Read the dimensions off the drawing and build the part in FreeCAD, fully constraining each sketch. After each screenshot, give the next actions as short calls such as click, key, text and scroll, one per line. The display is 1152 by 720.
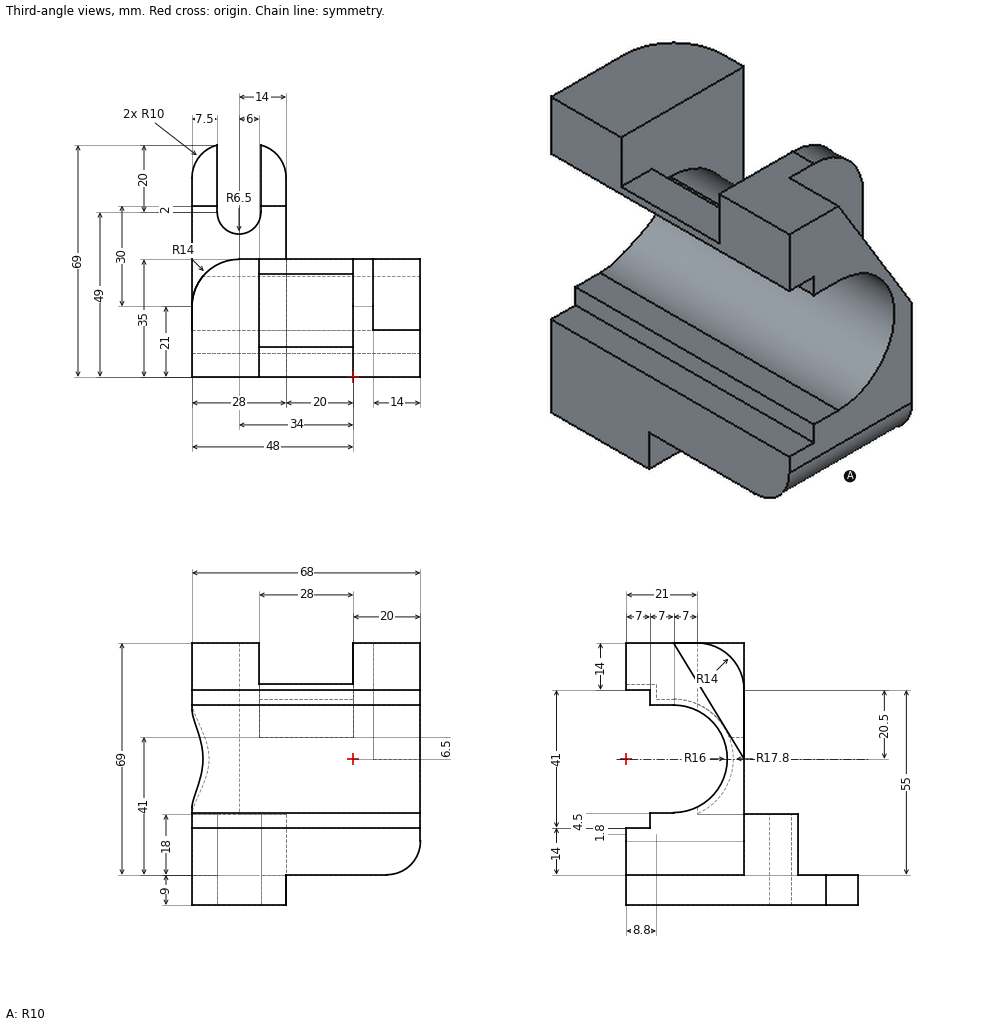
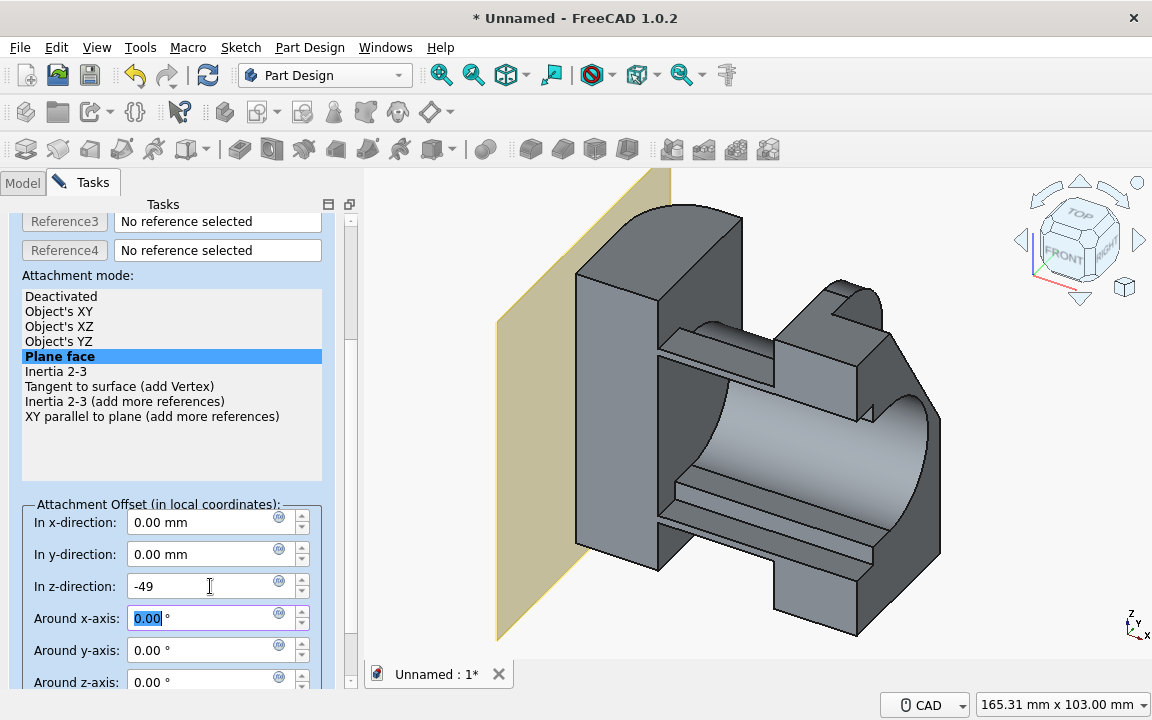
scroll(351, 451, up, 4)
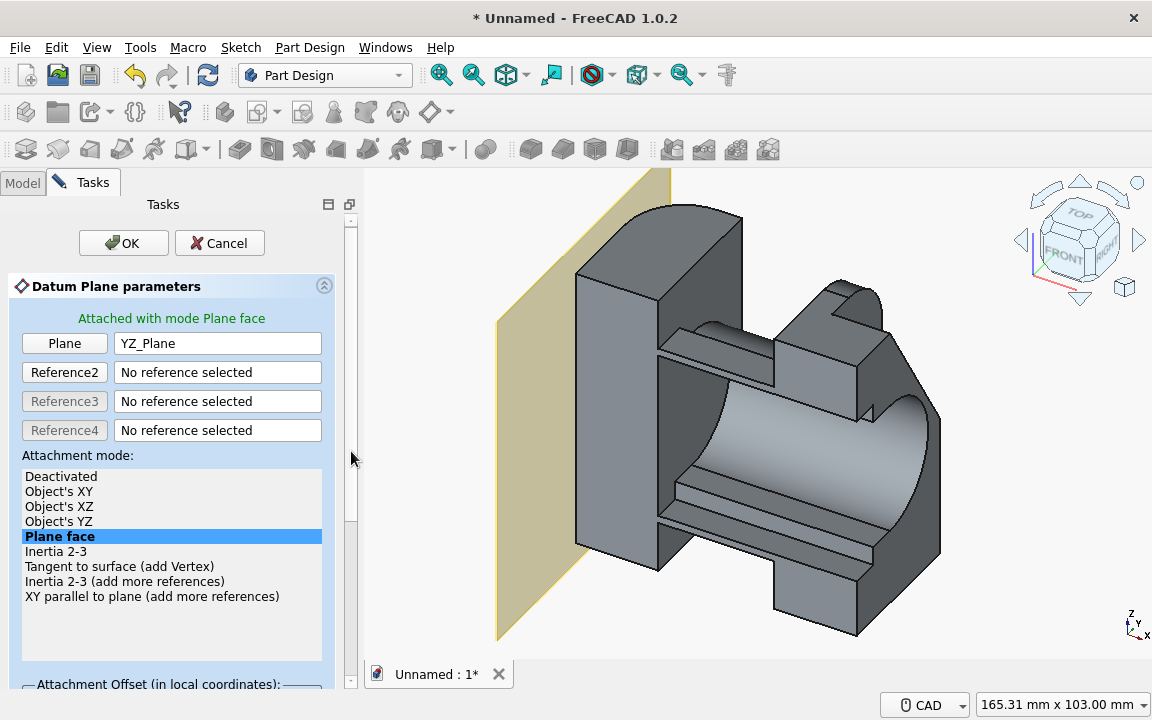
click(124, 243)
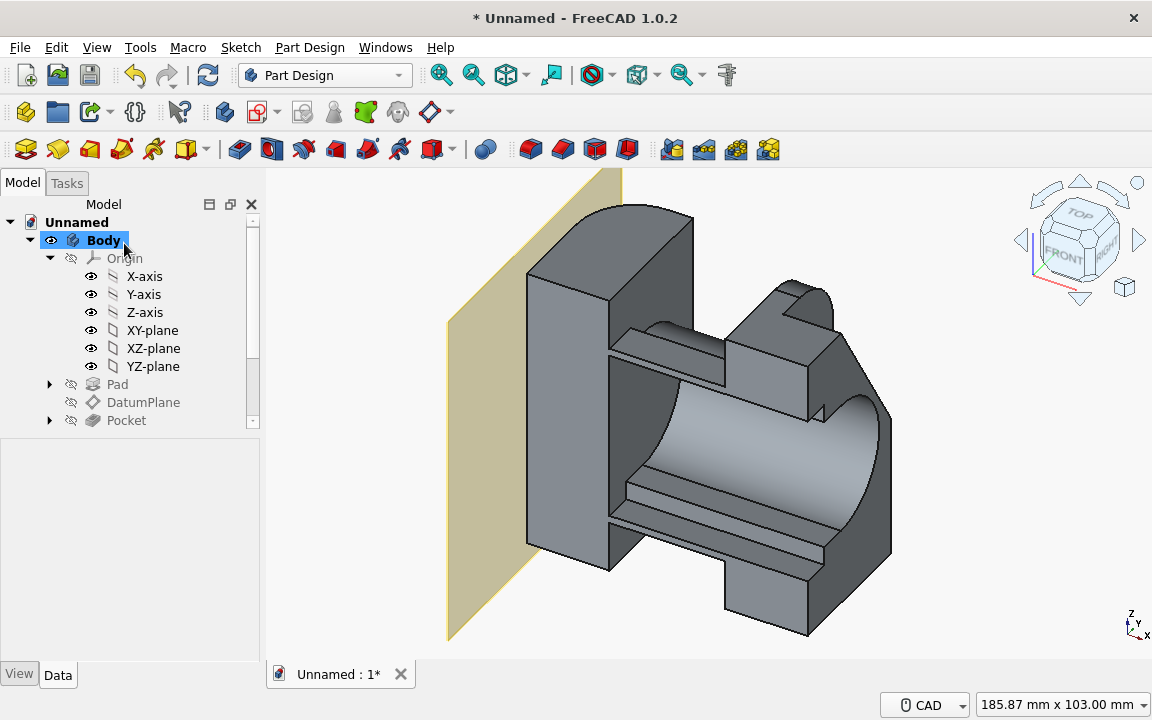
scroll(100, 326, down, 3)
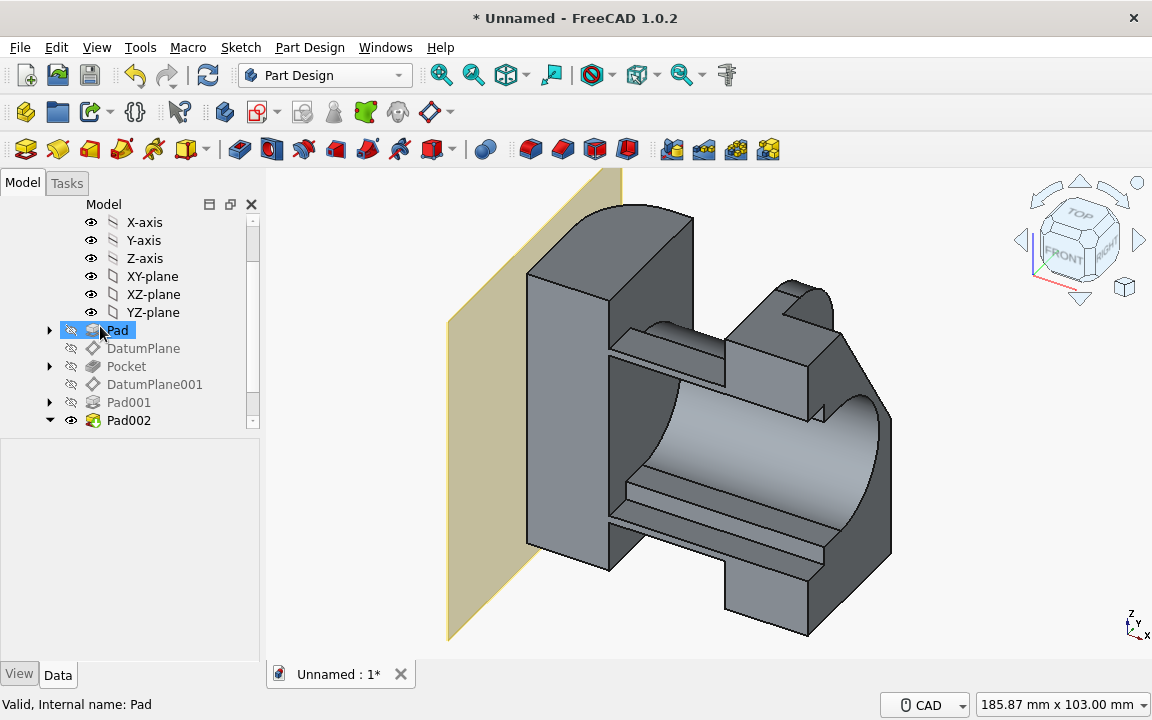
click(116, 420)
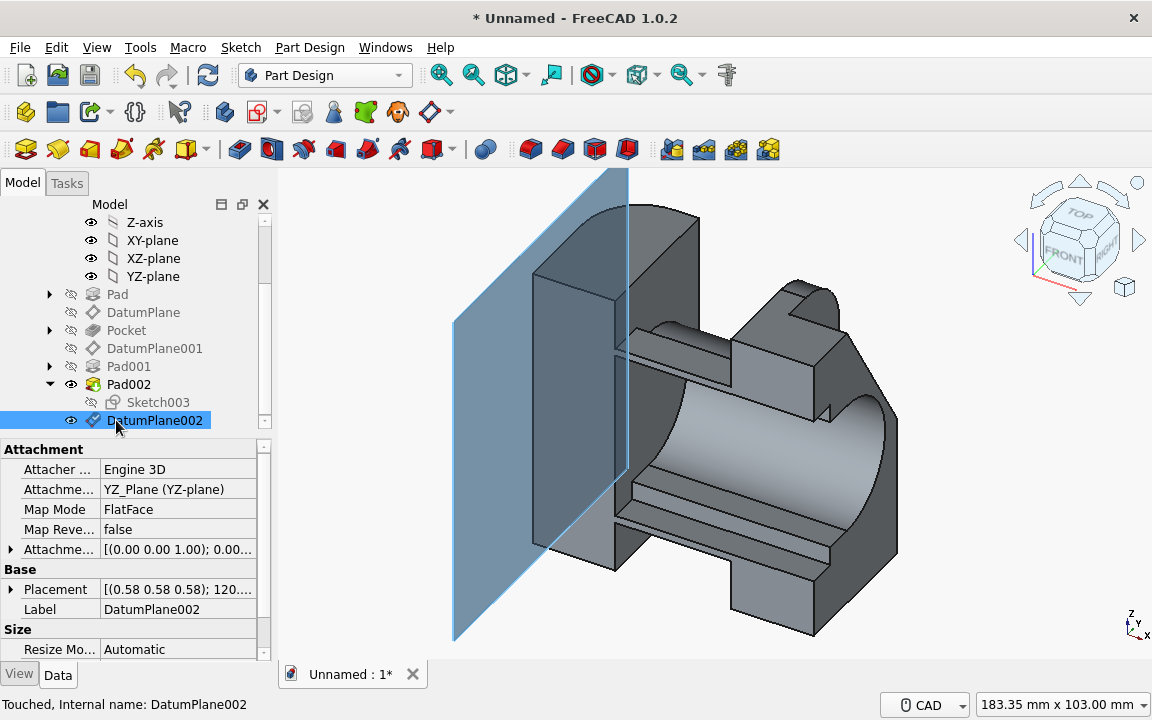
click(258, 112)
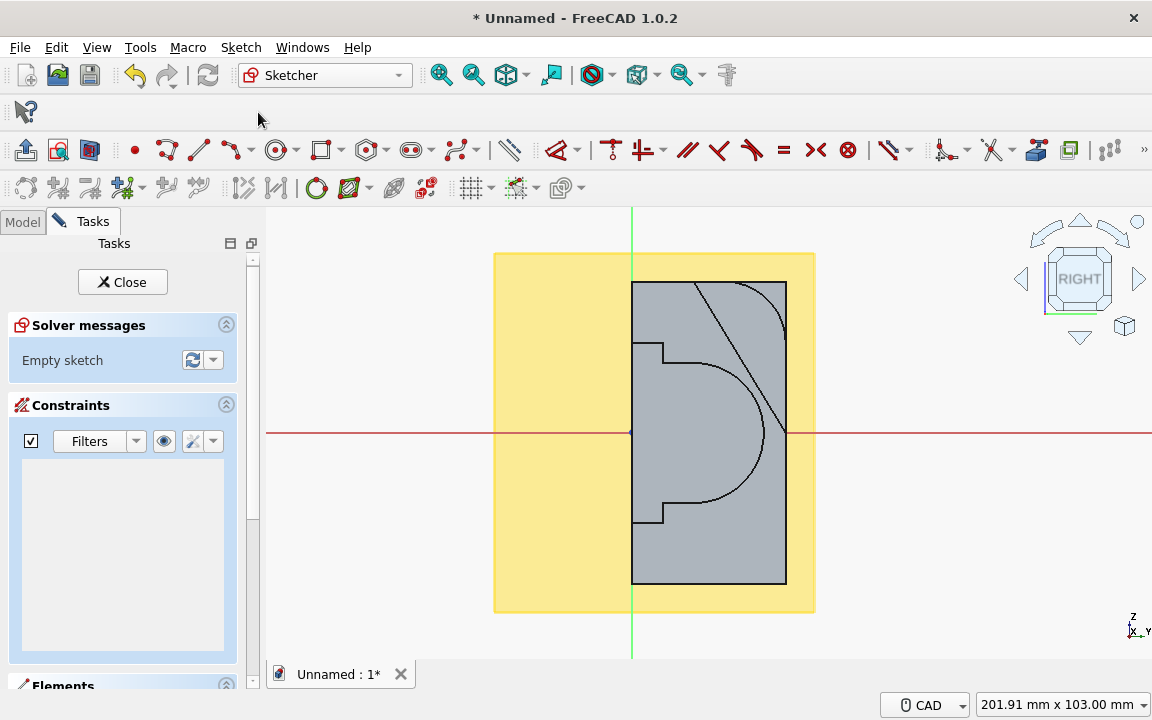
click(90, 150)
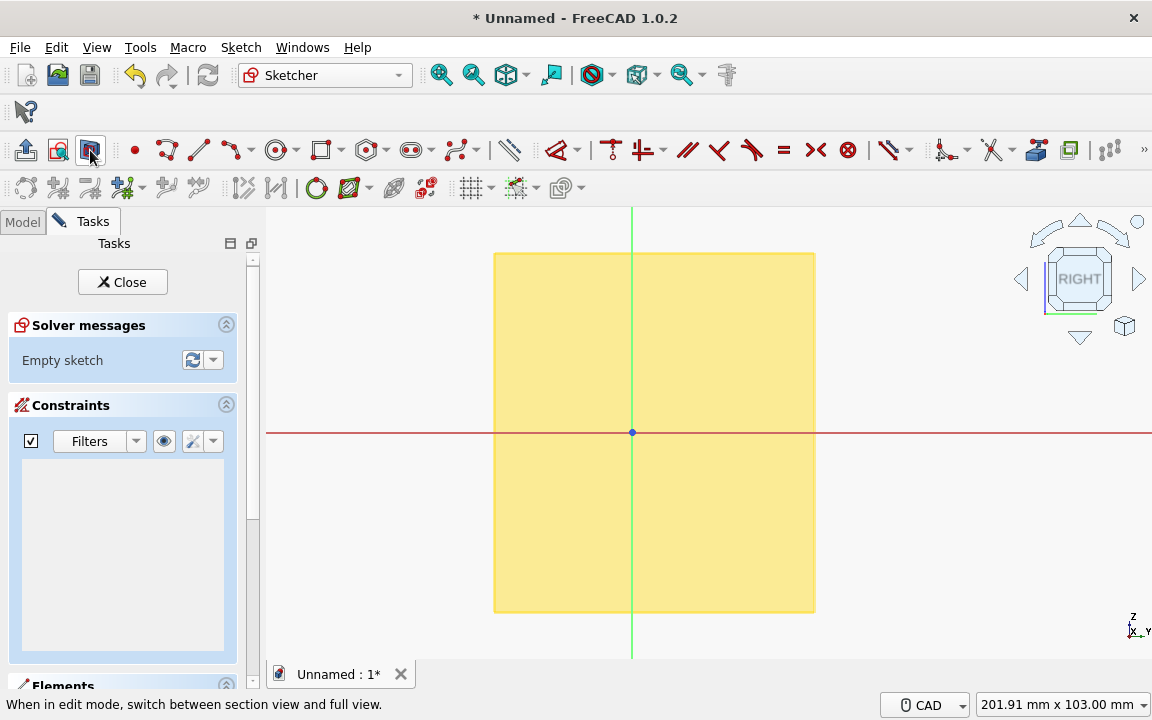
scroll(815, 433, up, 2)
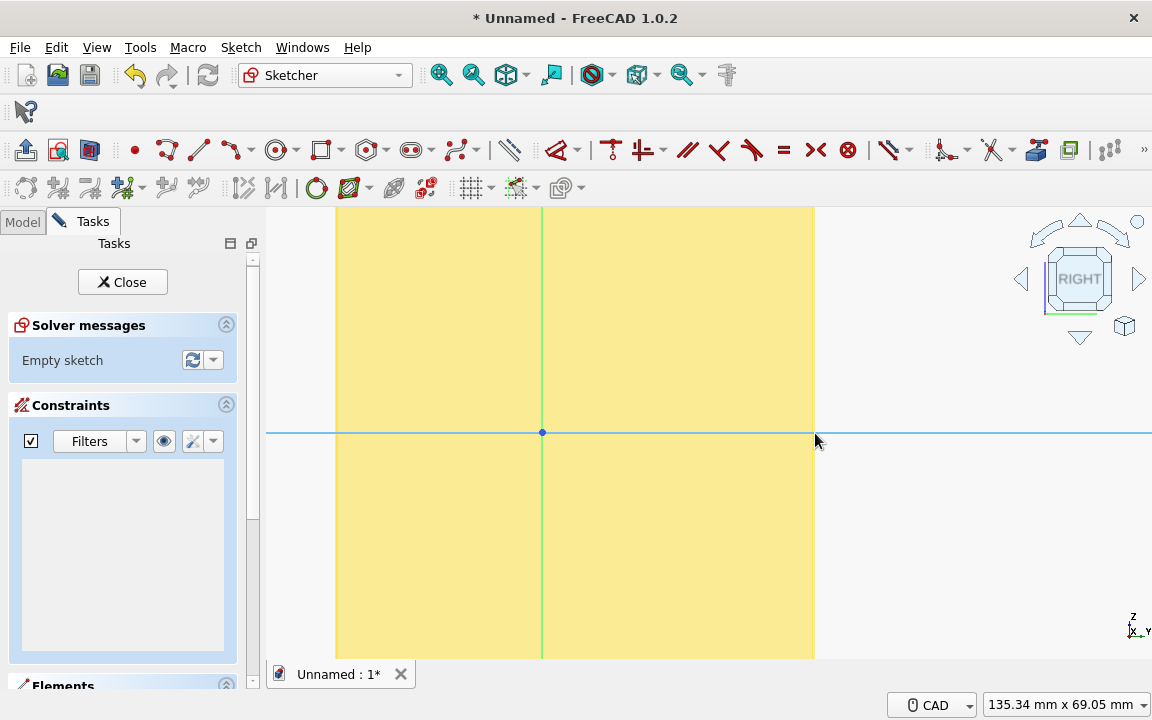
click(168, 150)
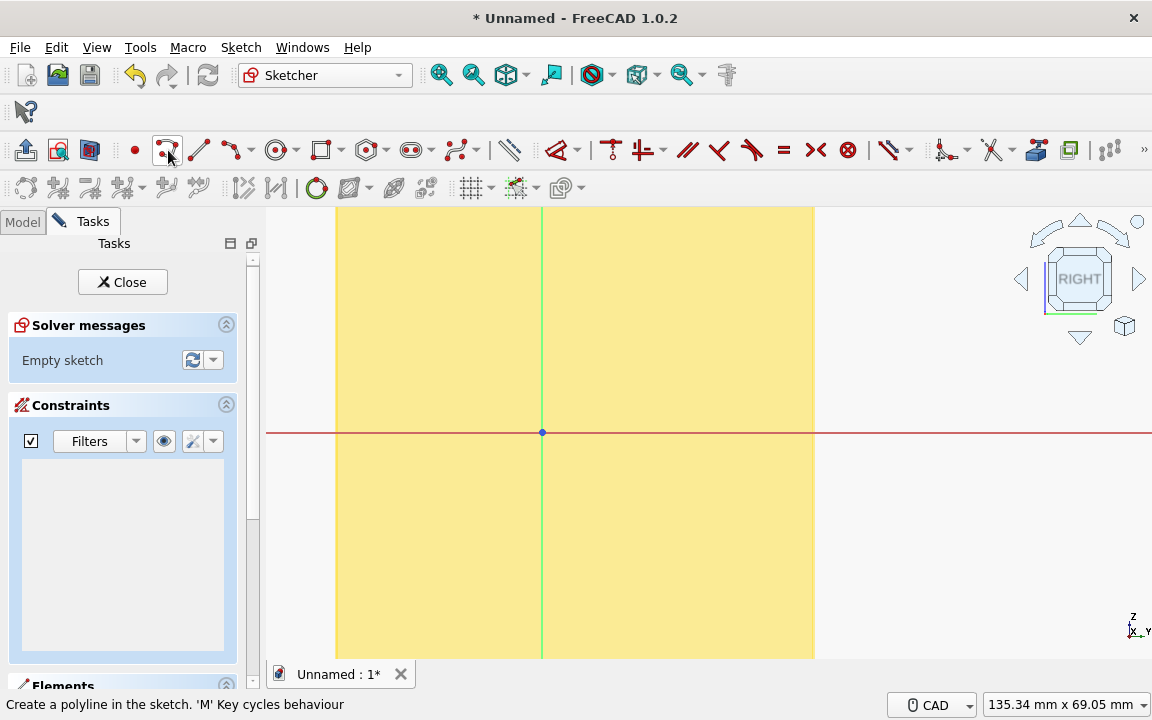
click(634, 328)
click(588, 328)
click(588, 299)
click(542, 299)
click(551, 567)
click(588, 567)
click(588, 537)
click(634, 537)
right_click(634, 537)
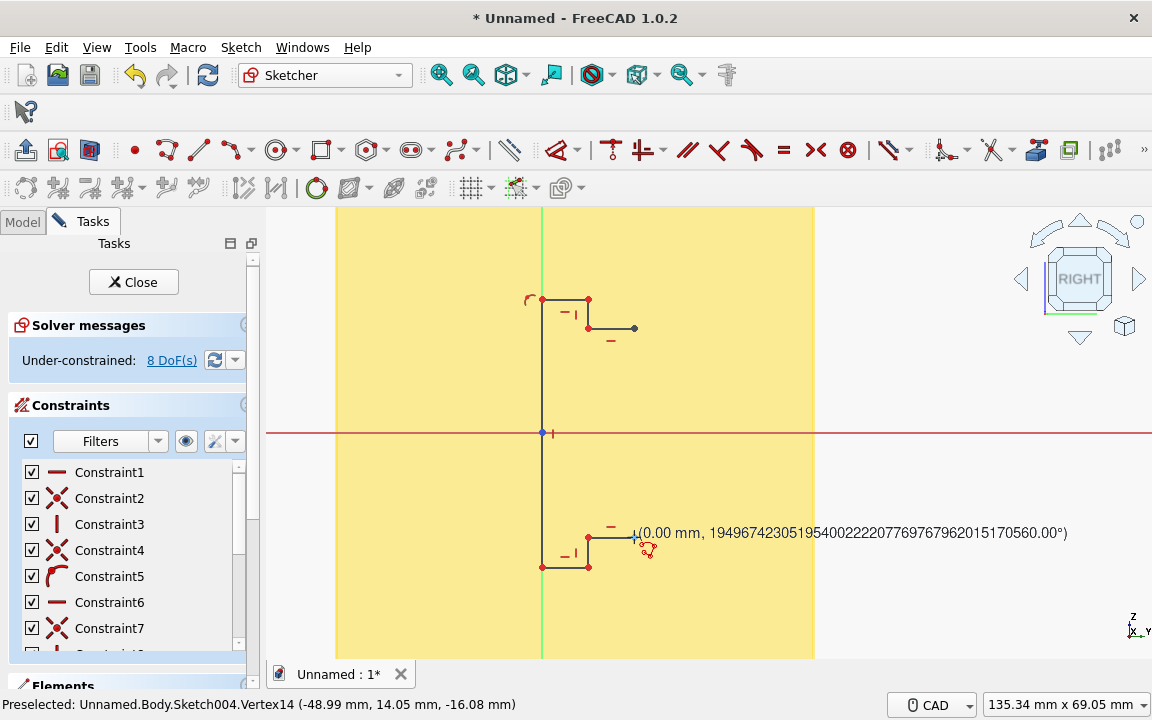
key(g)
key(3)
key(a)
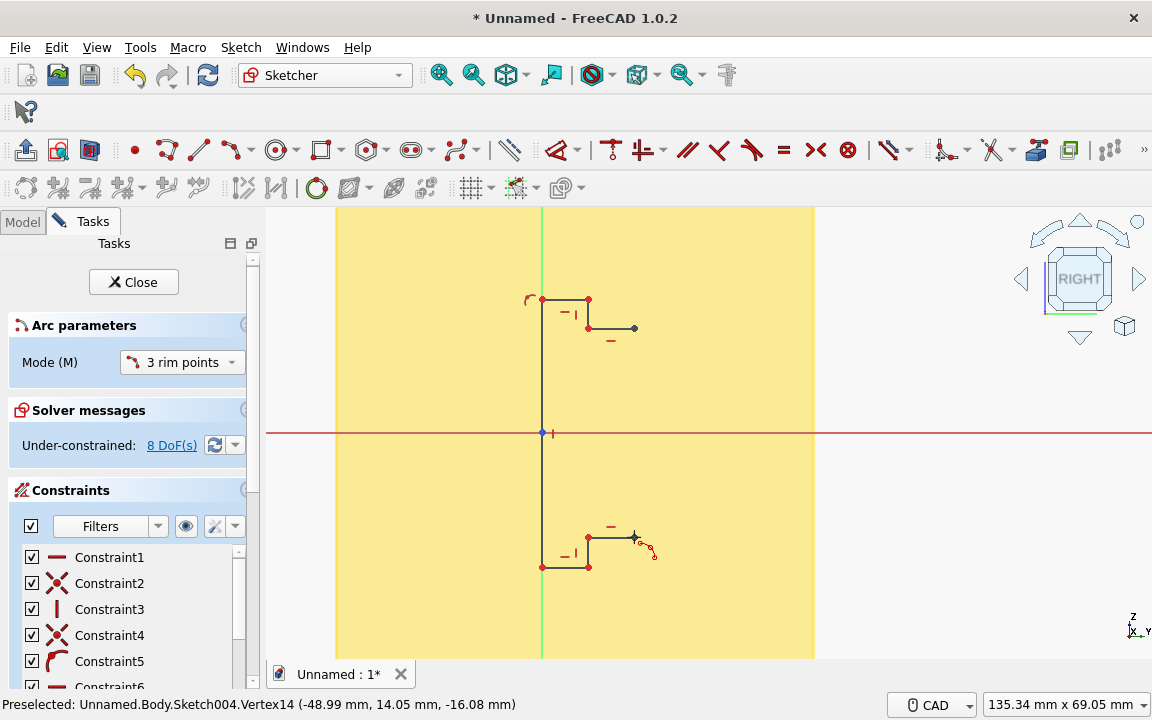
click(634, 538)
click(634, 329)
click(733, 465)
key(Escape)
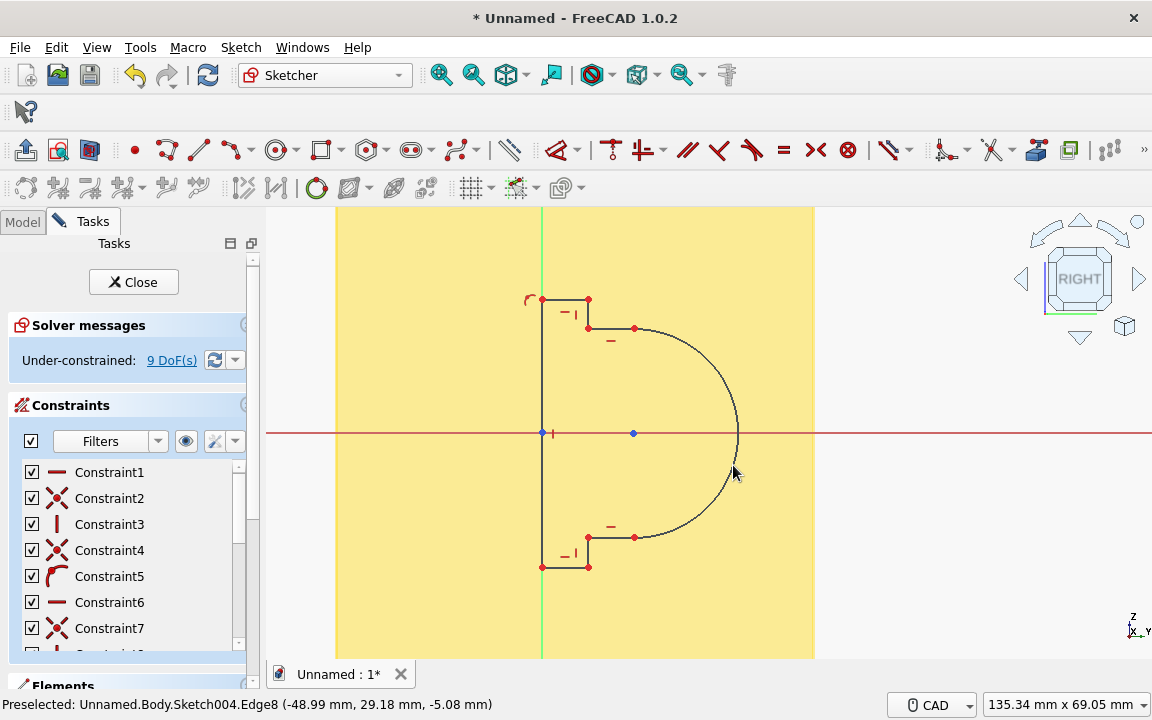
click(620, 329)